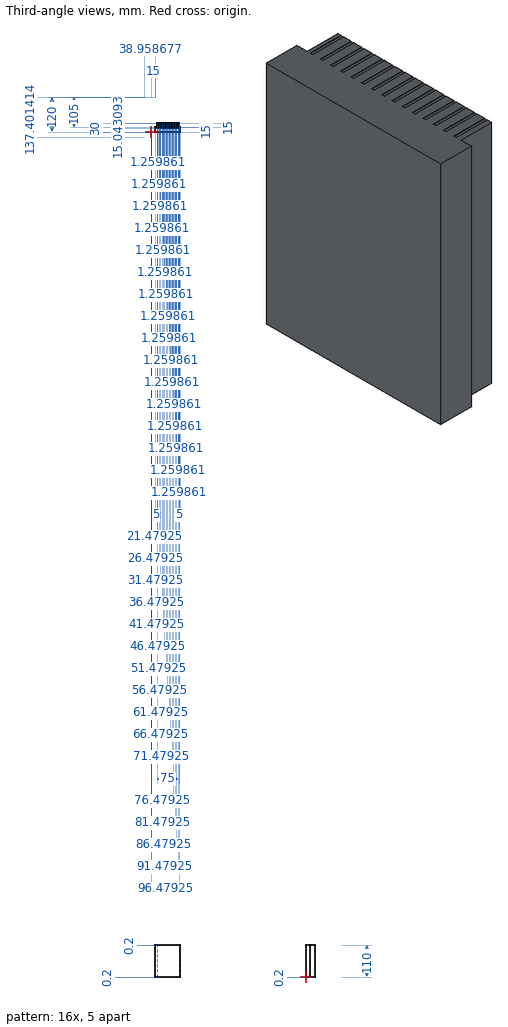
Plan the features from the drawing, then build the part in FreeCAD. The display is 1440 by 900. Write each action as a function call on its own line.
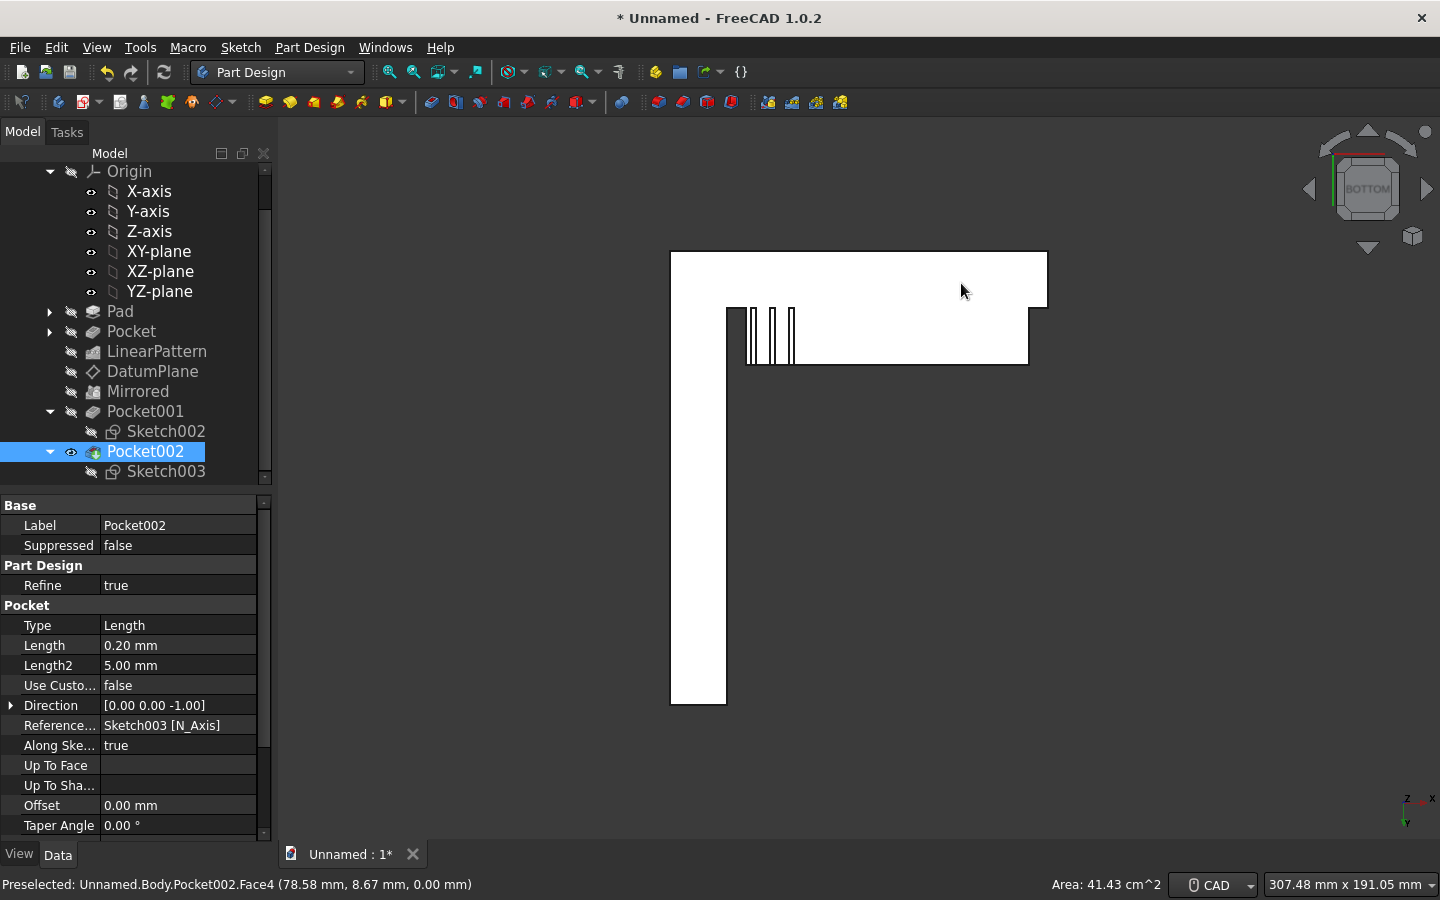
click(84, 102)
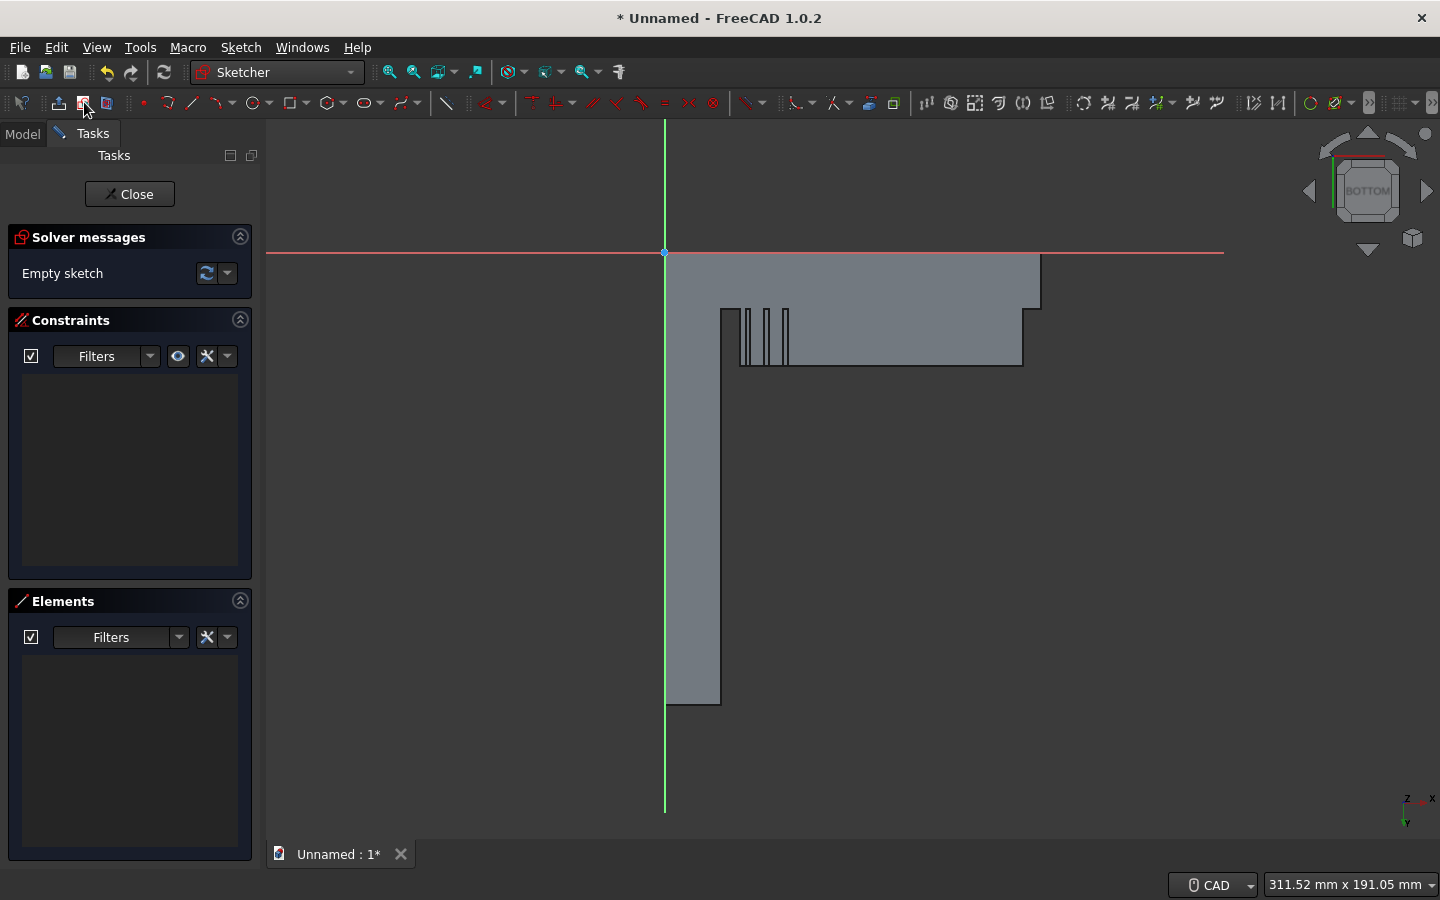
scroll(807, 320, up, 11)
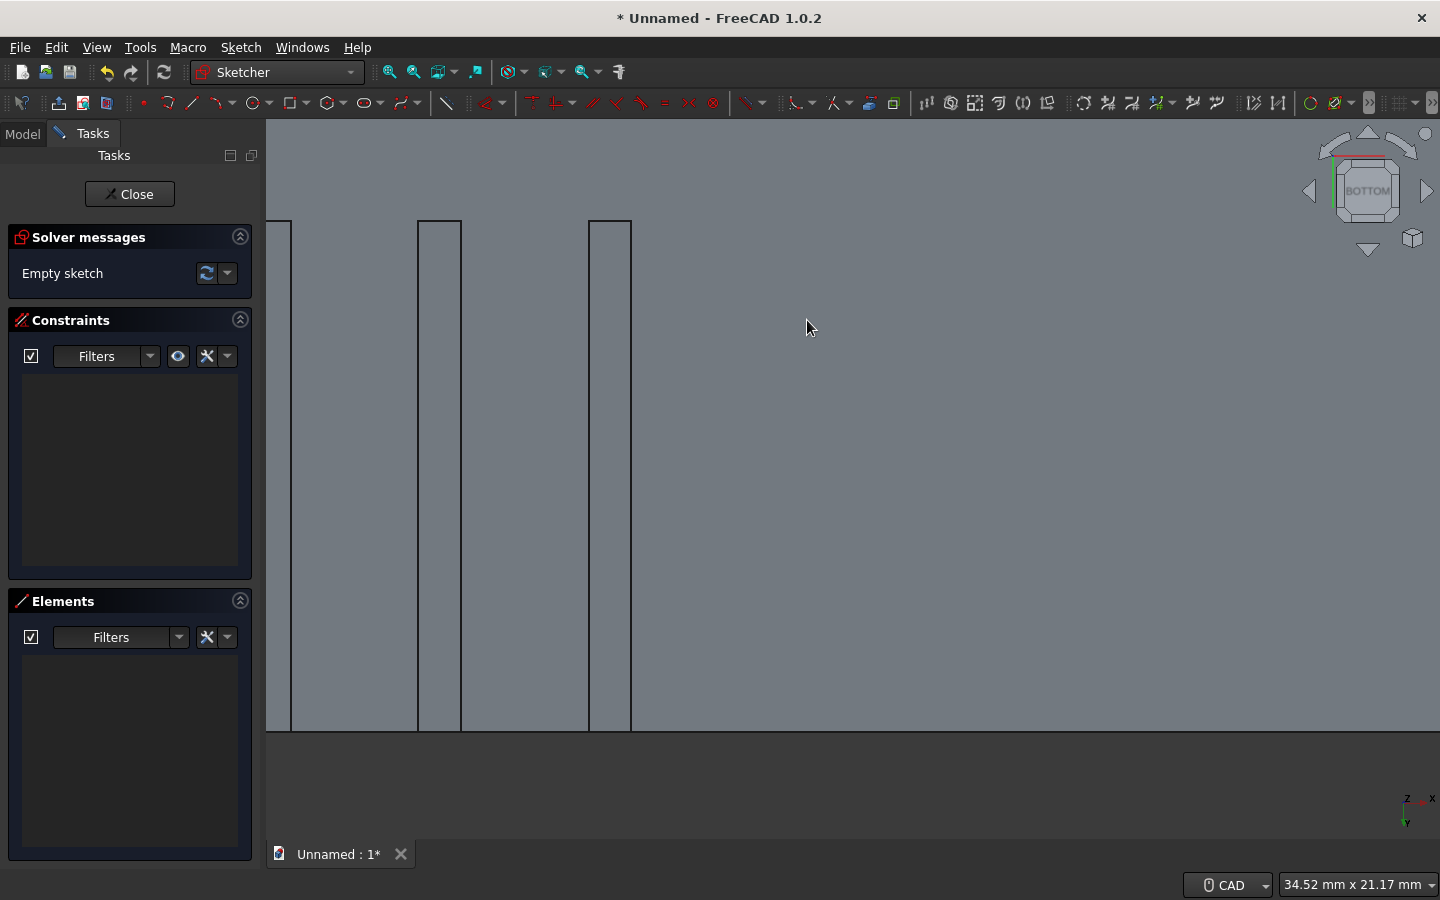
click(290, 104)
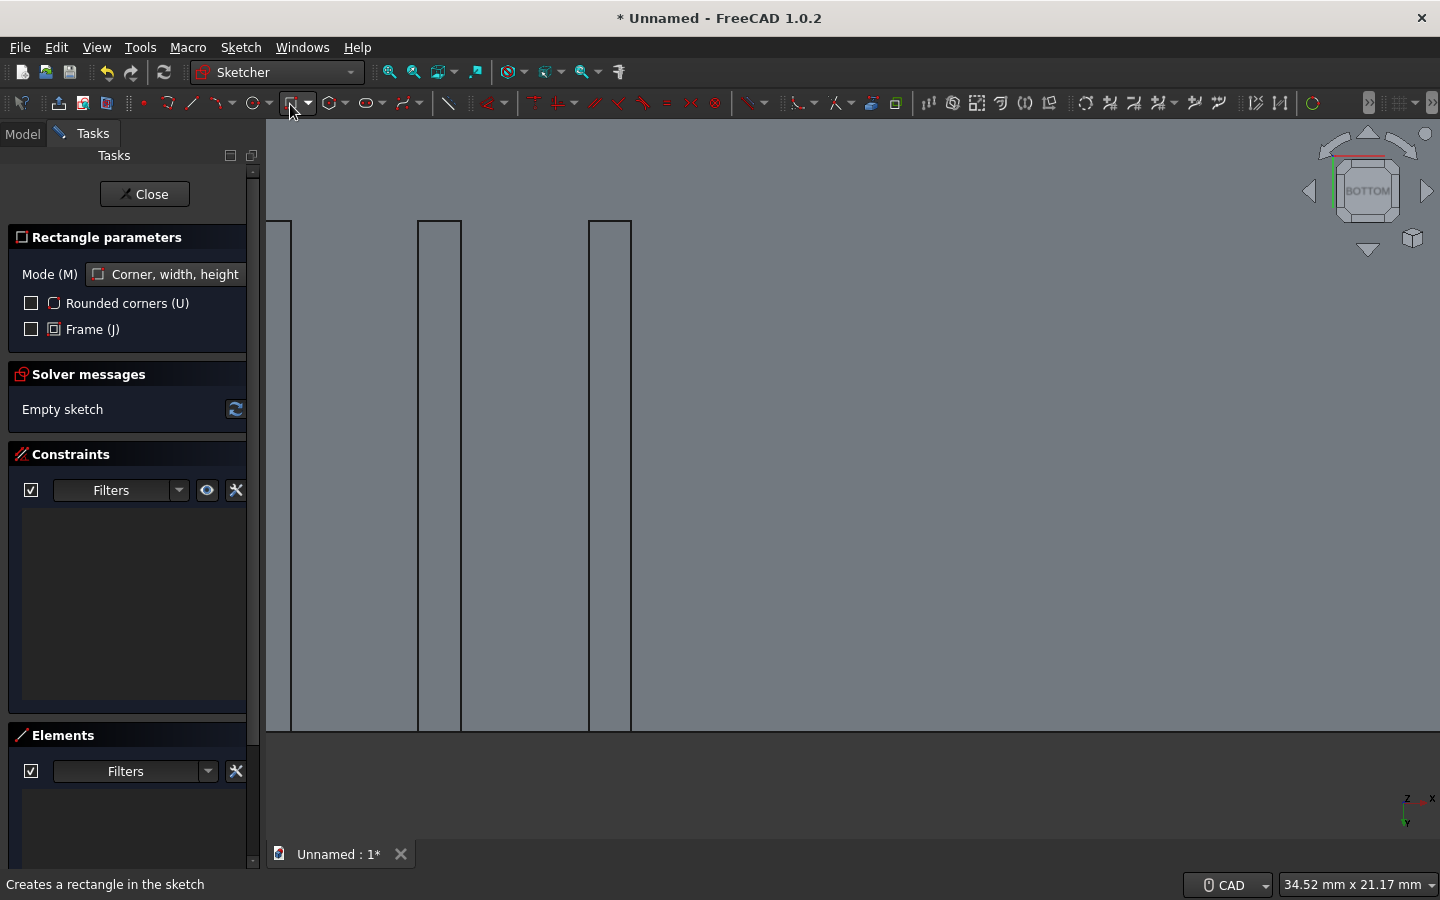
click(759, 221)
click(801, 732)
key(Escape)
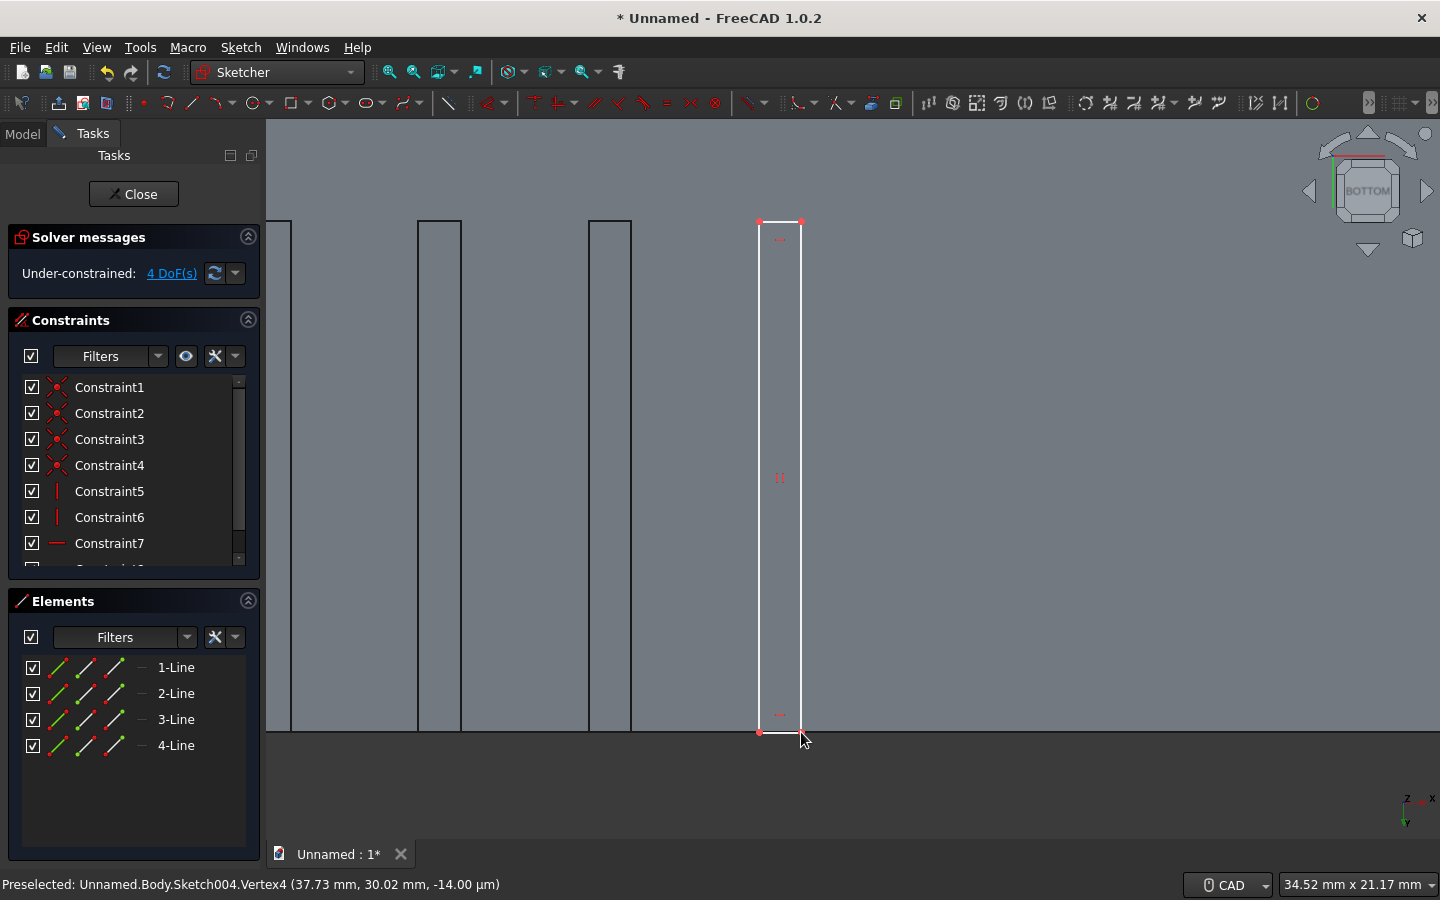
click(488, 104)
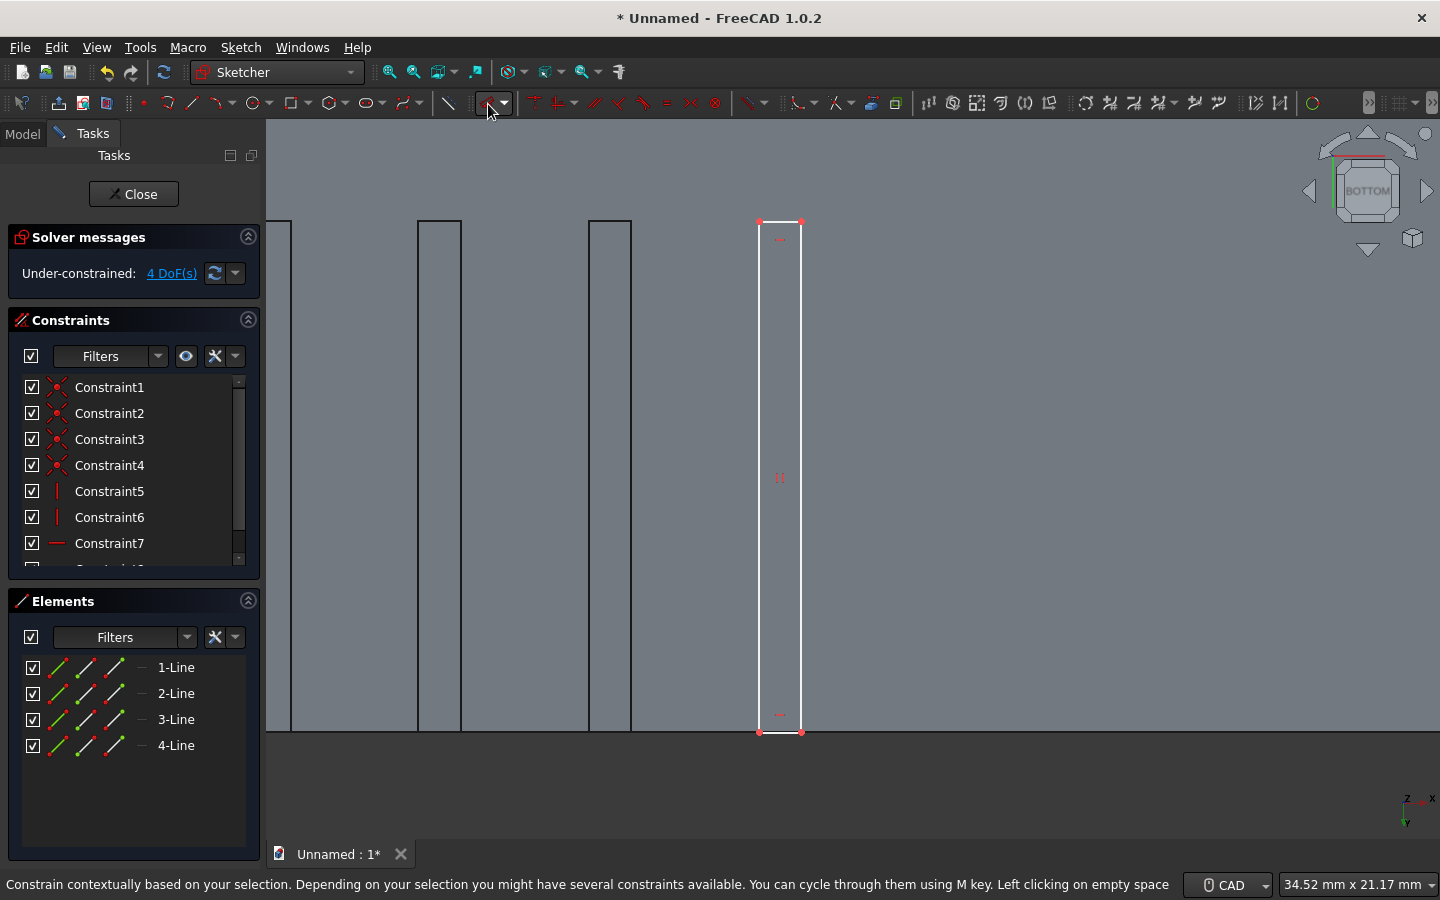
click(759, 733)
click(817, 440)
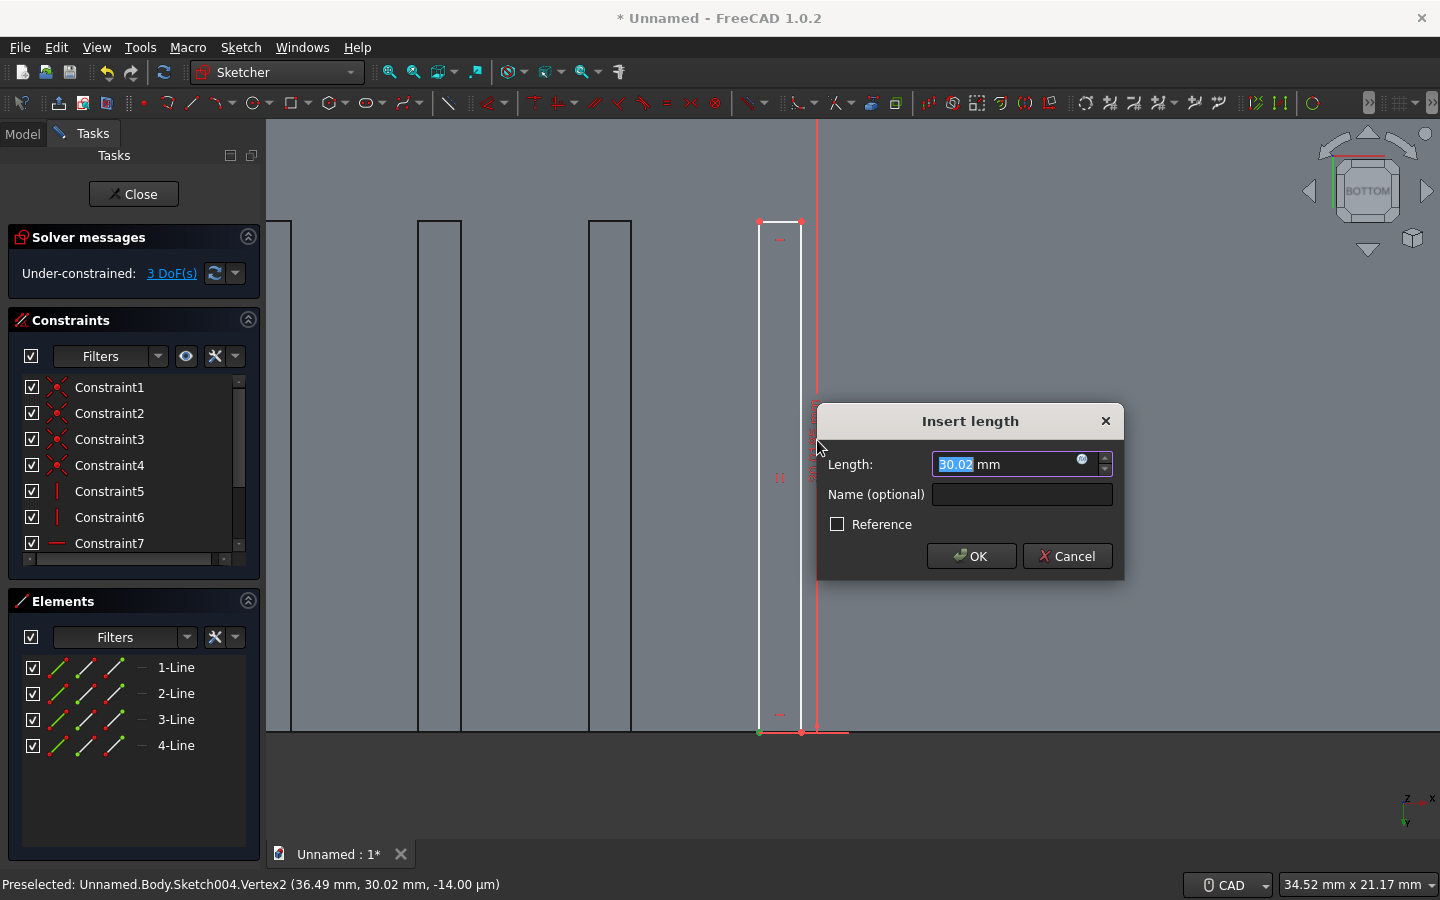
text(30)
key(Return)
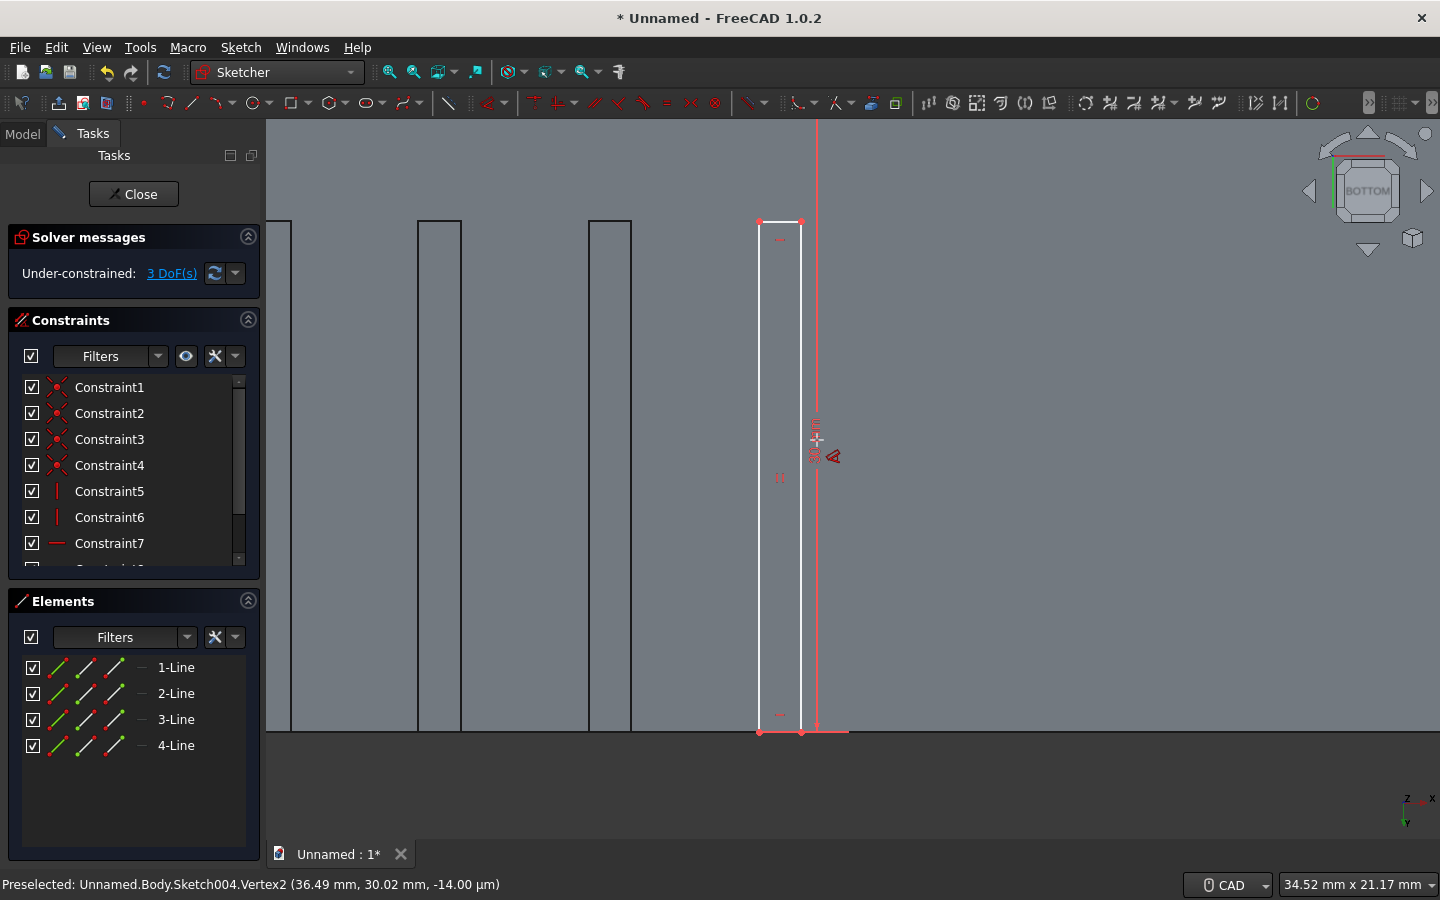
click(772, 732)
click(780, 766)